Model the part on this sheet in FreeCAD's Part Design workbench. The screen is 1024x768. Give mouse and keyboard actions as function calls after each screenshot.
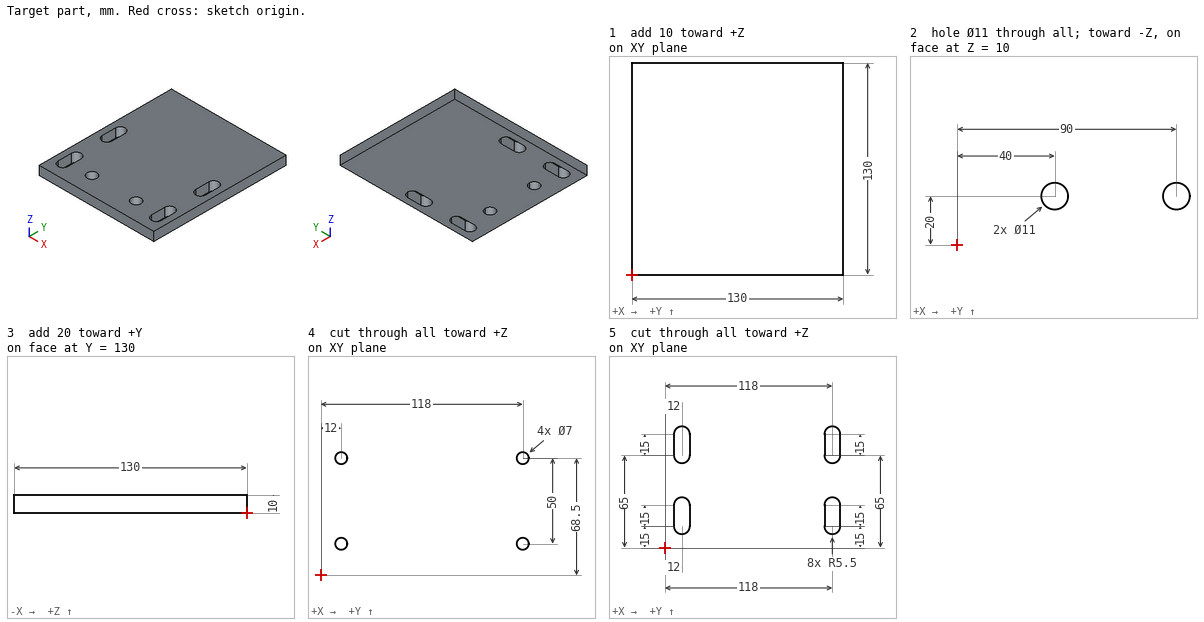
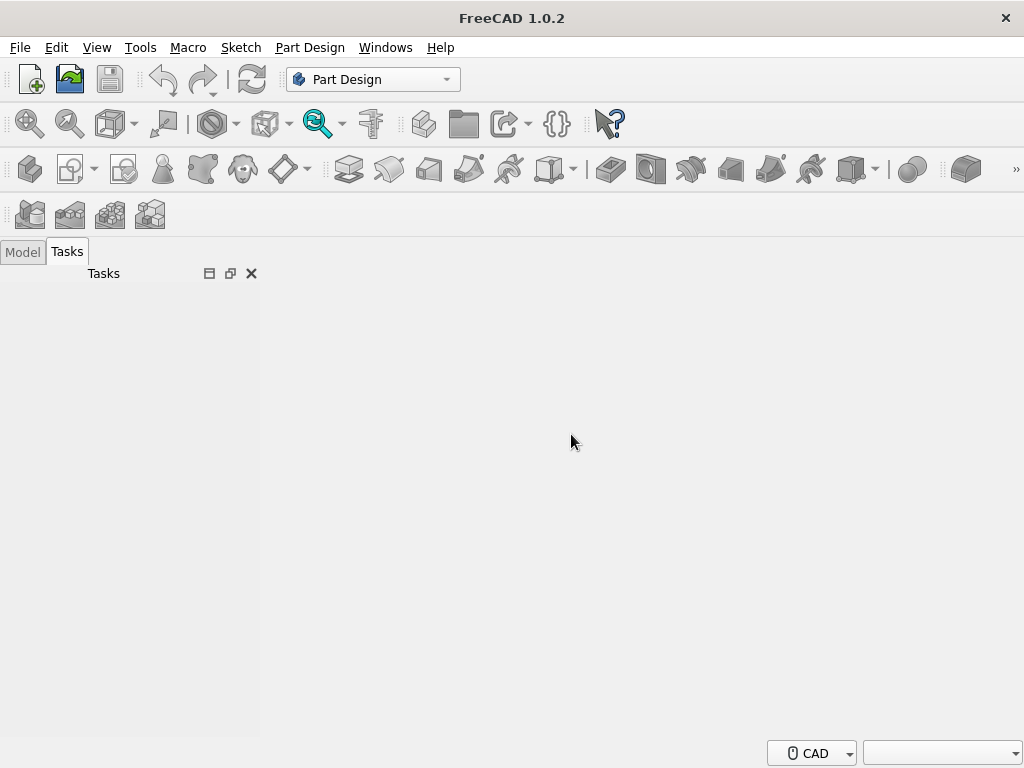
click(30, 80)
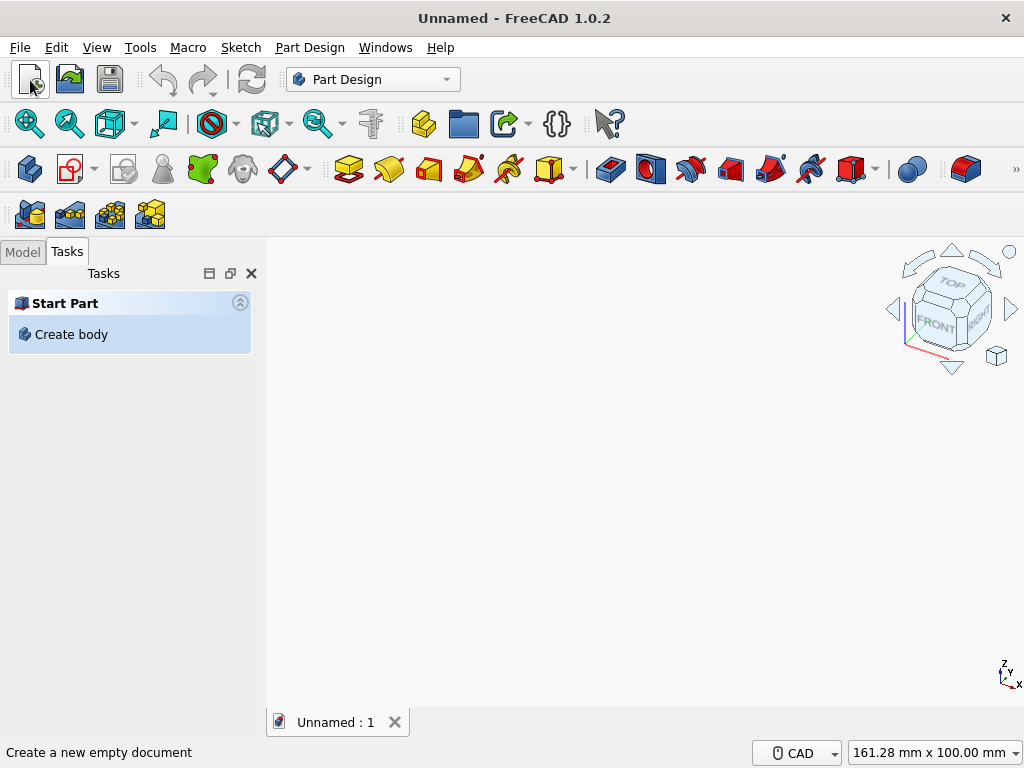
click(70, 170)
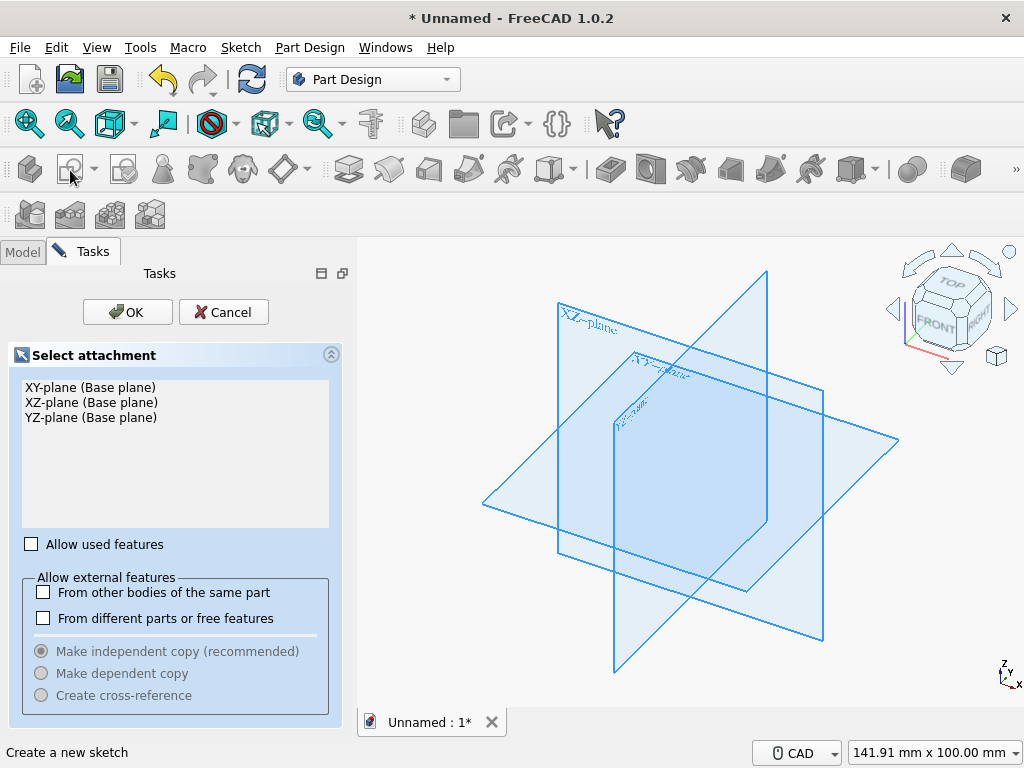
click(82, 388)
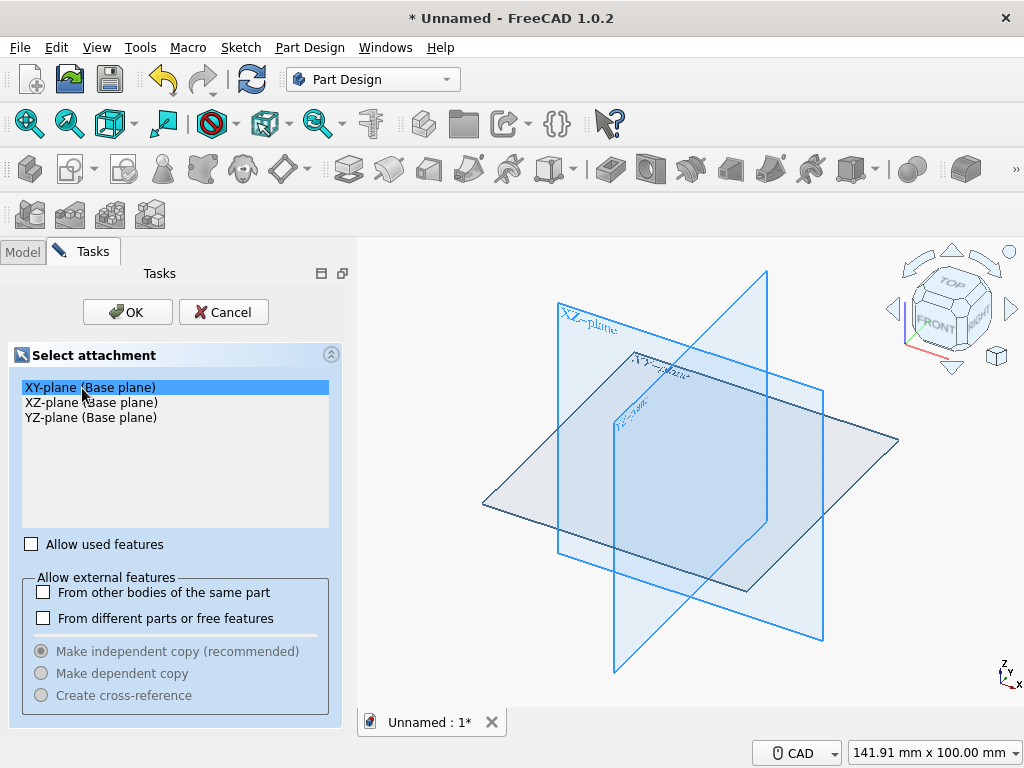
click(128, 312)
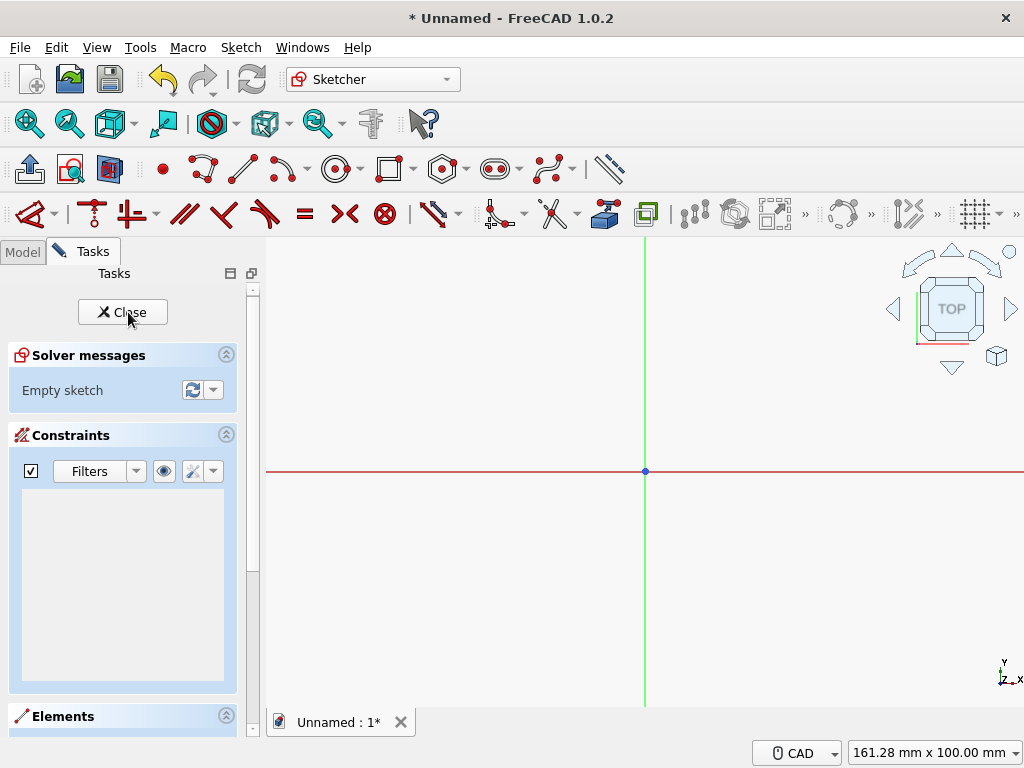
scroll(294, 679, down, 4)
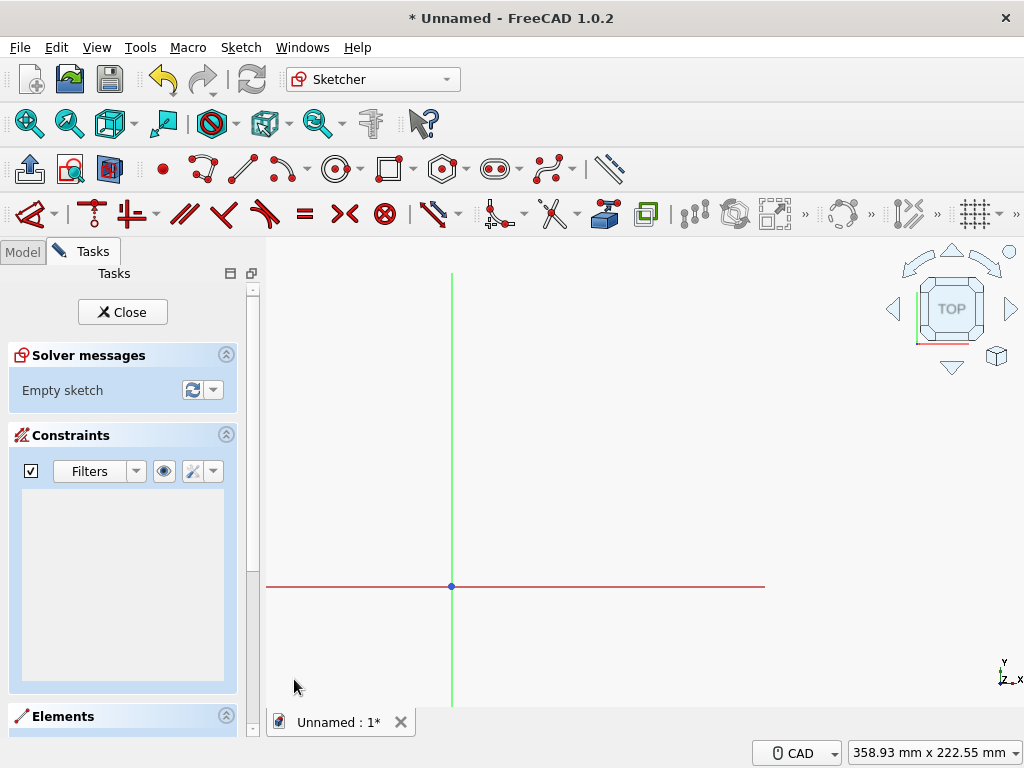
click(390, 170)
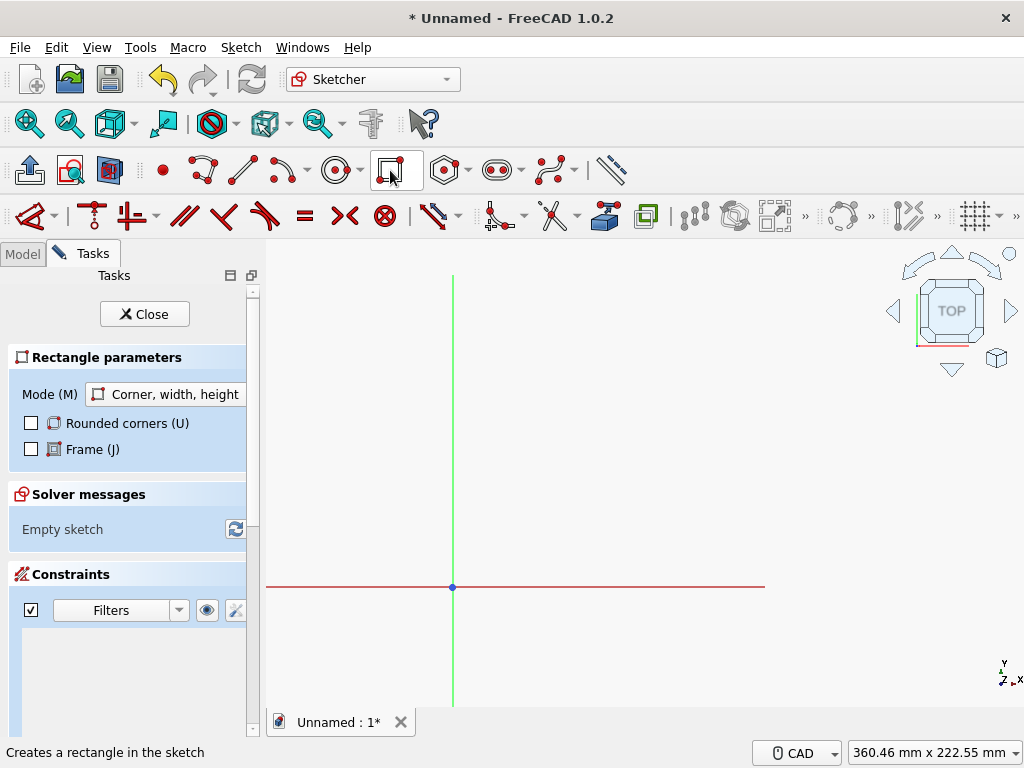
click(453, 587)
click(726, 314)
key(Escape)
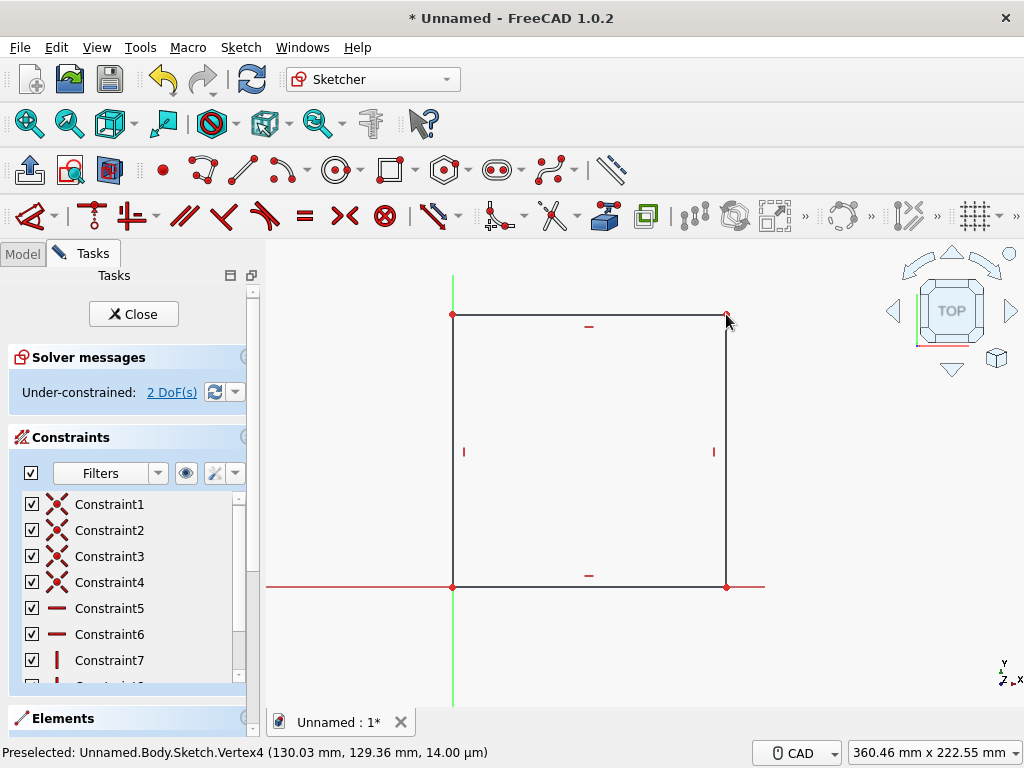
click(535, 587)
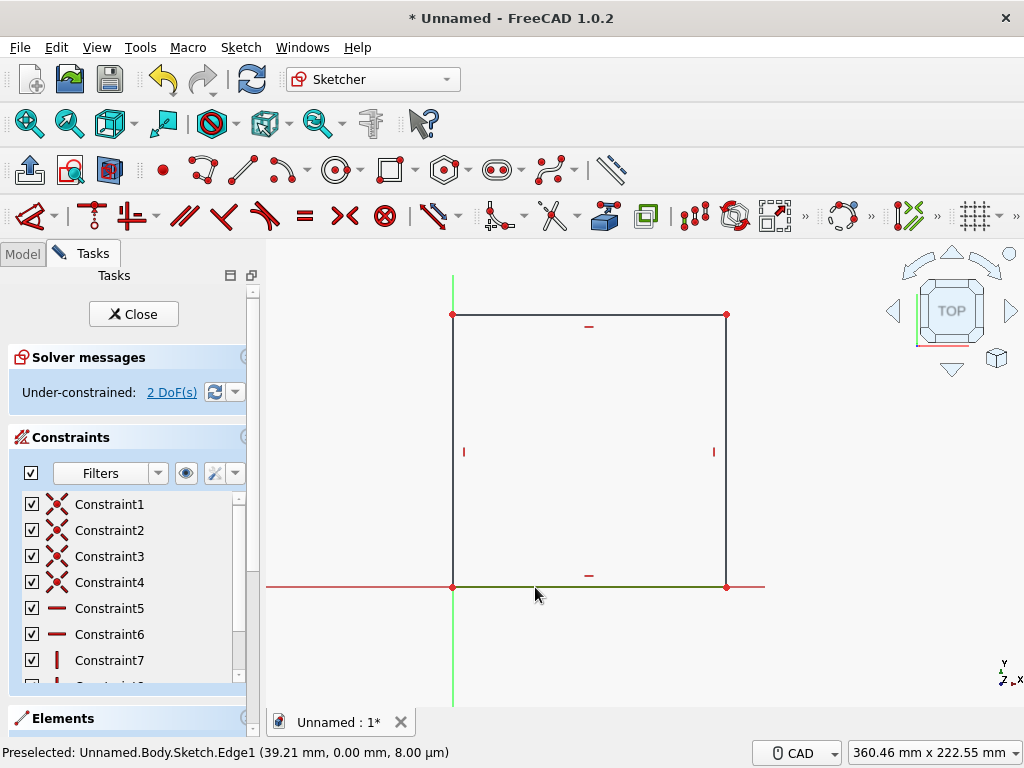
click(56, 216)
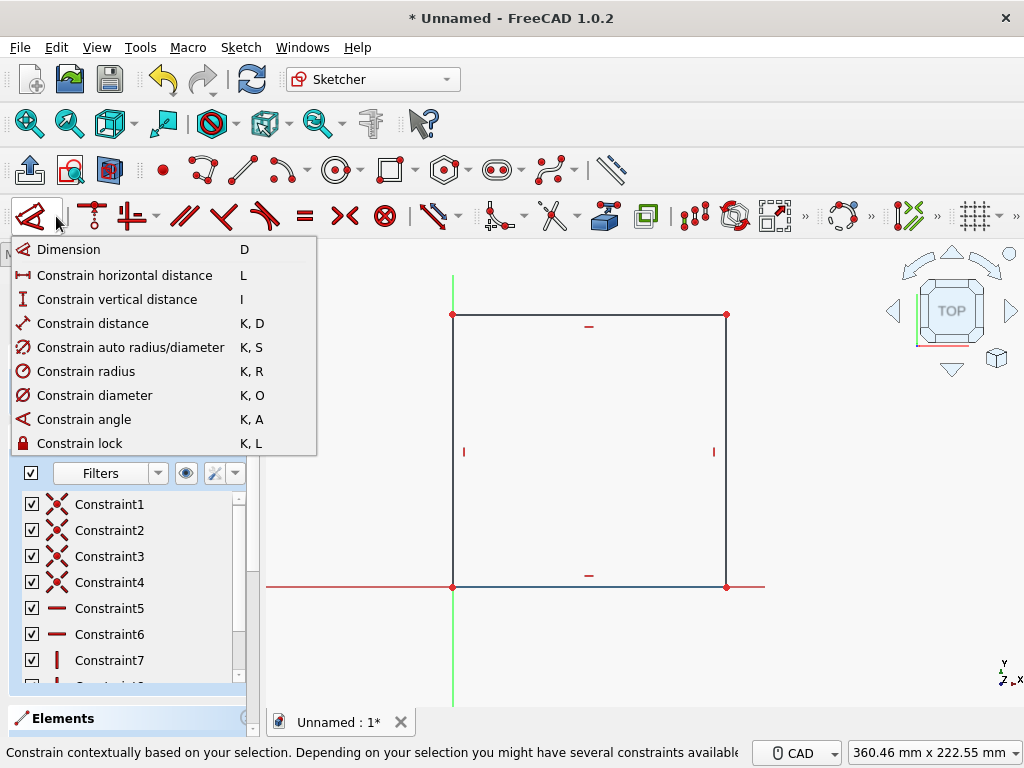
click(164, 275)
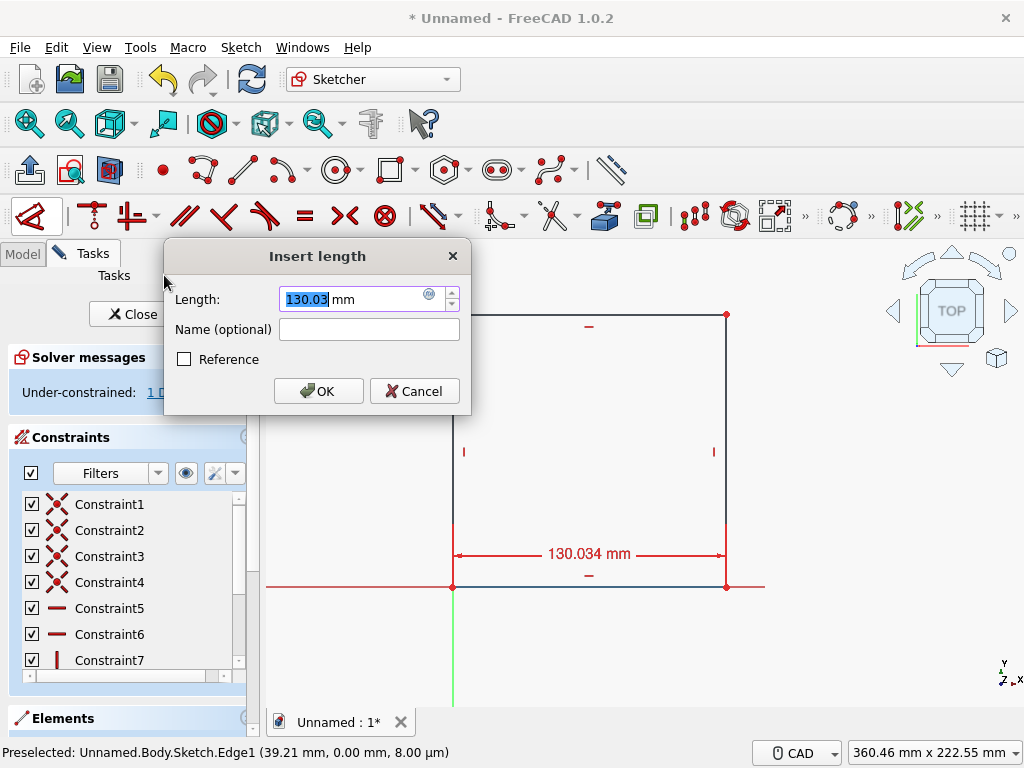
text(130)
key(Return)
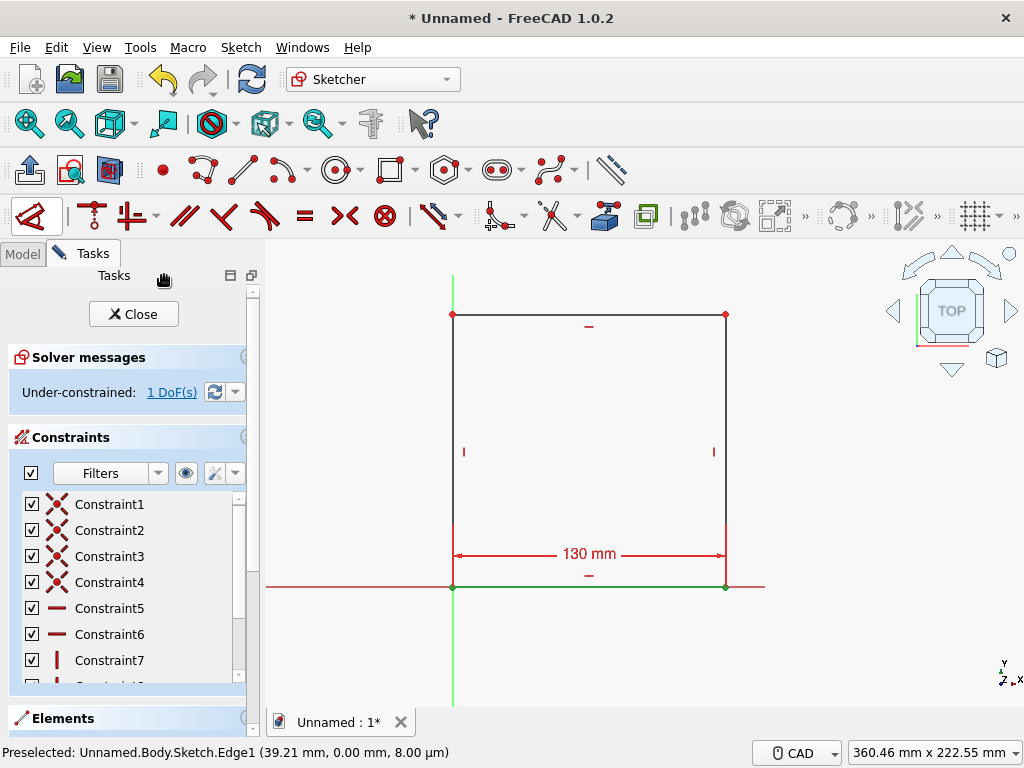
click(726, 505)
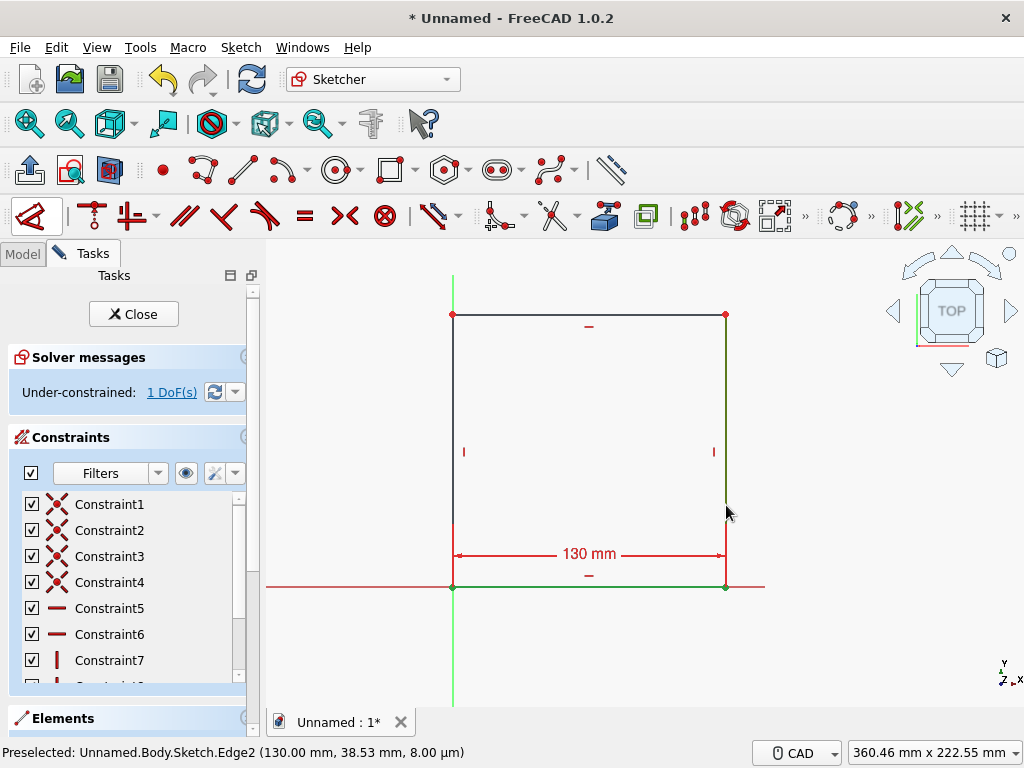
click(56, 216)